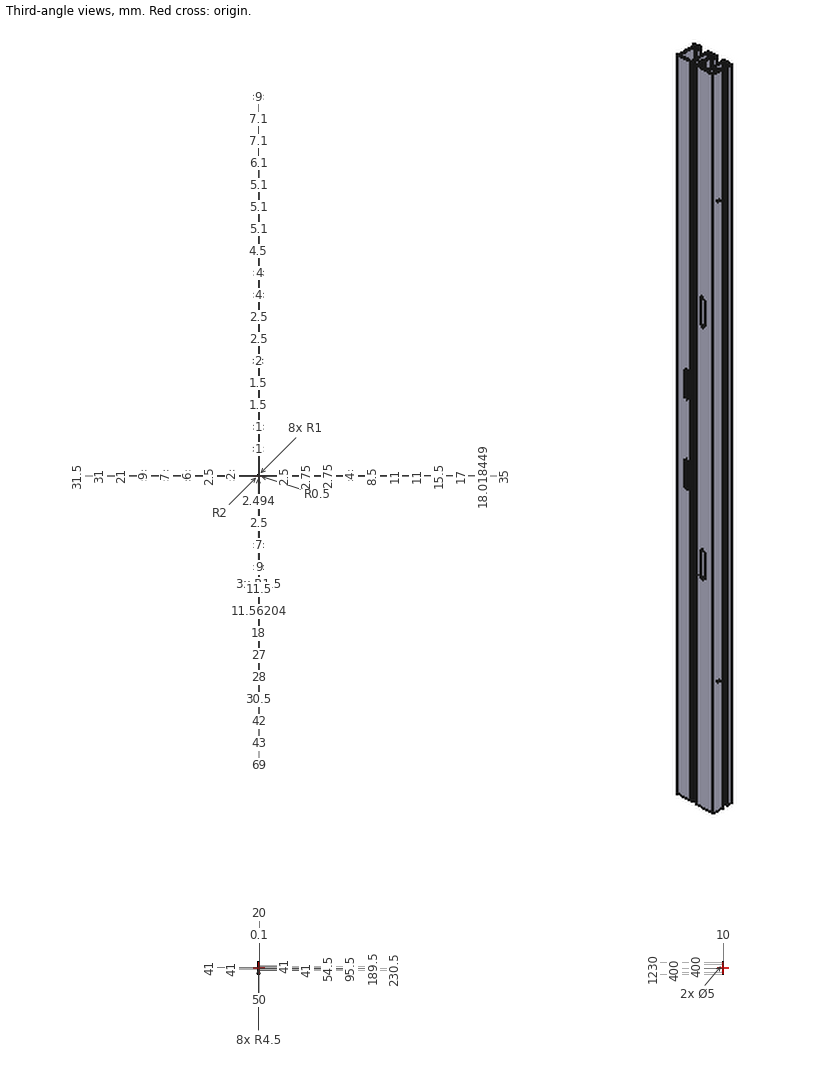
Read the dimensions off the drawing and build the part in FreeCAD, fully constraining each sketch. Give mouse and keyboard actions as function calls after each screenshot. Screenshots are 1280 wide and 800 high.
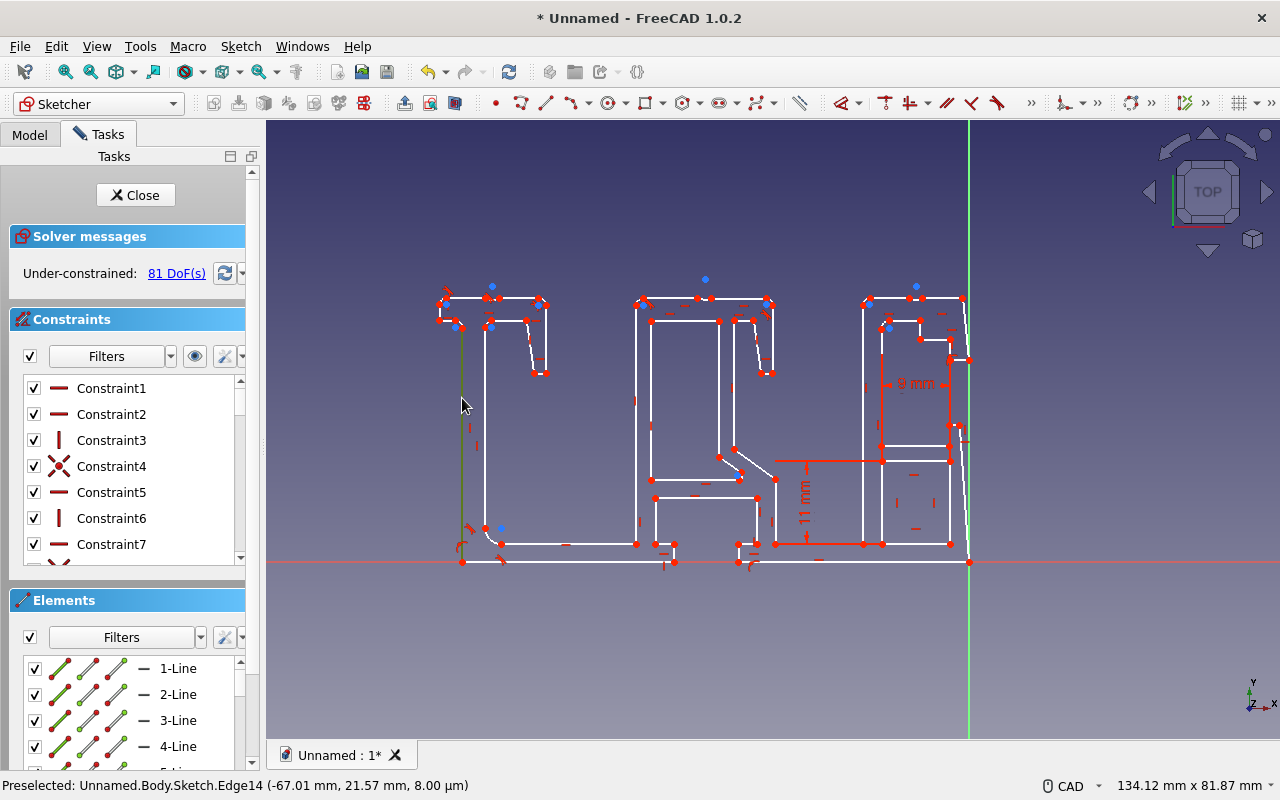
scroll(461, 323, up, 5)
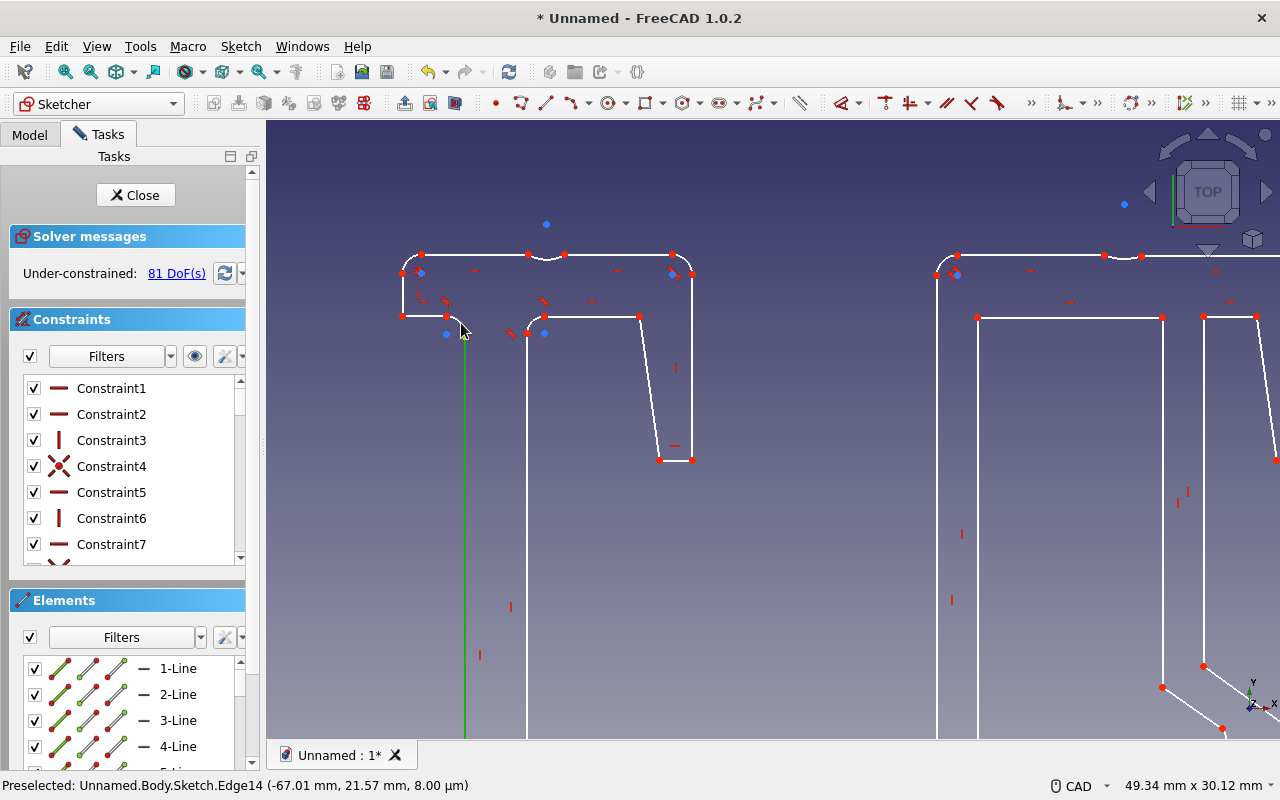
click(460, 323)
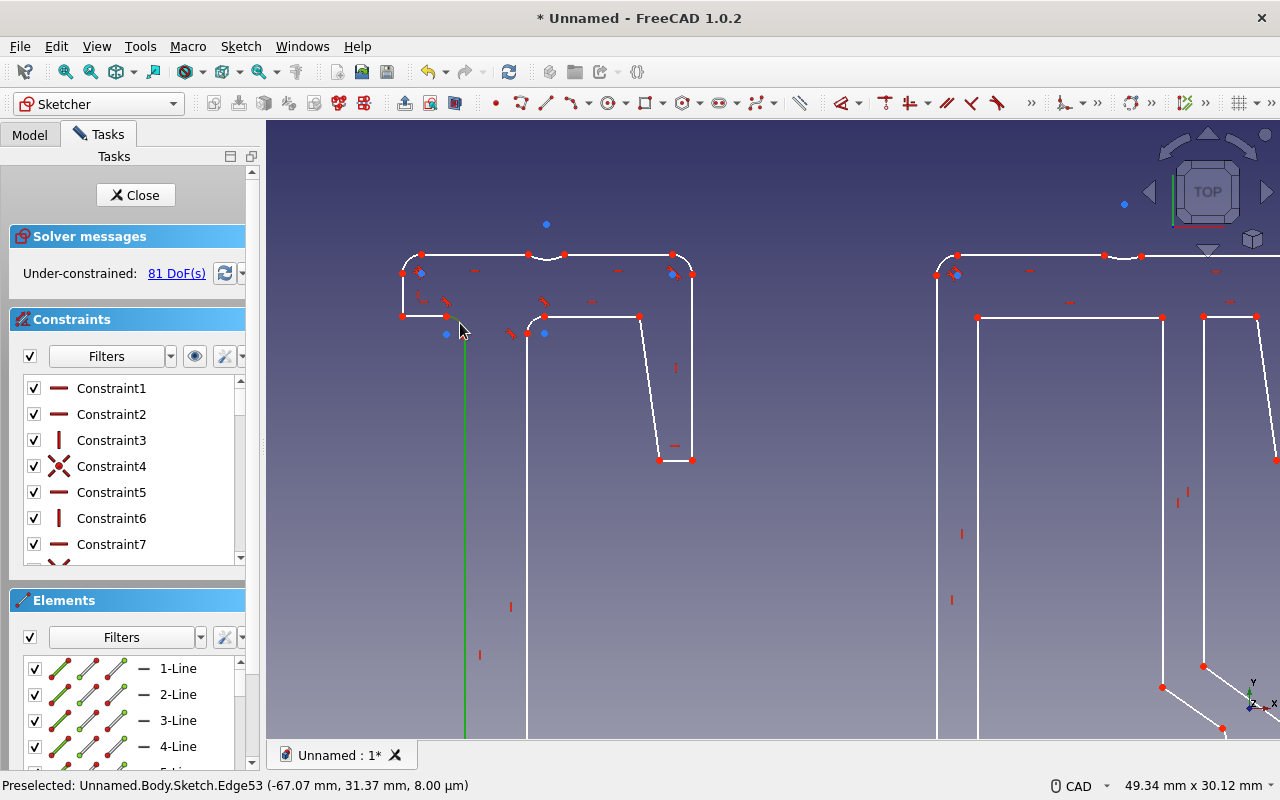
click(997, 104)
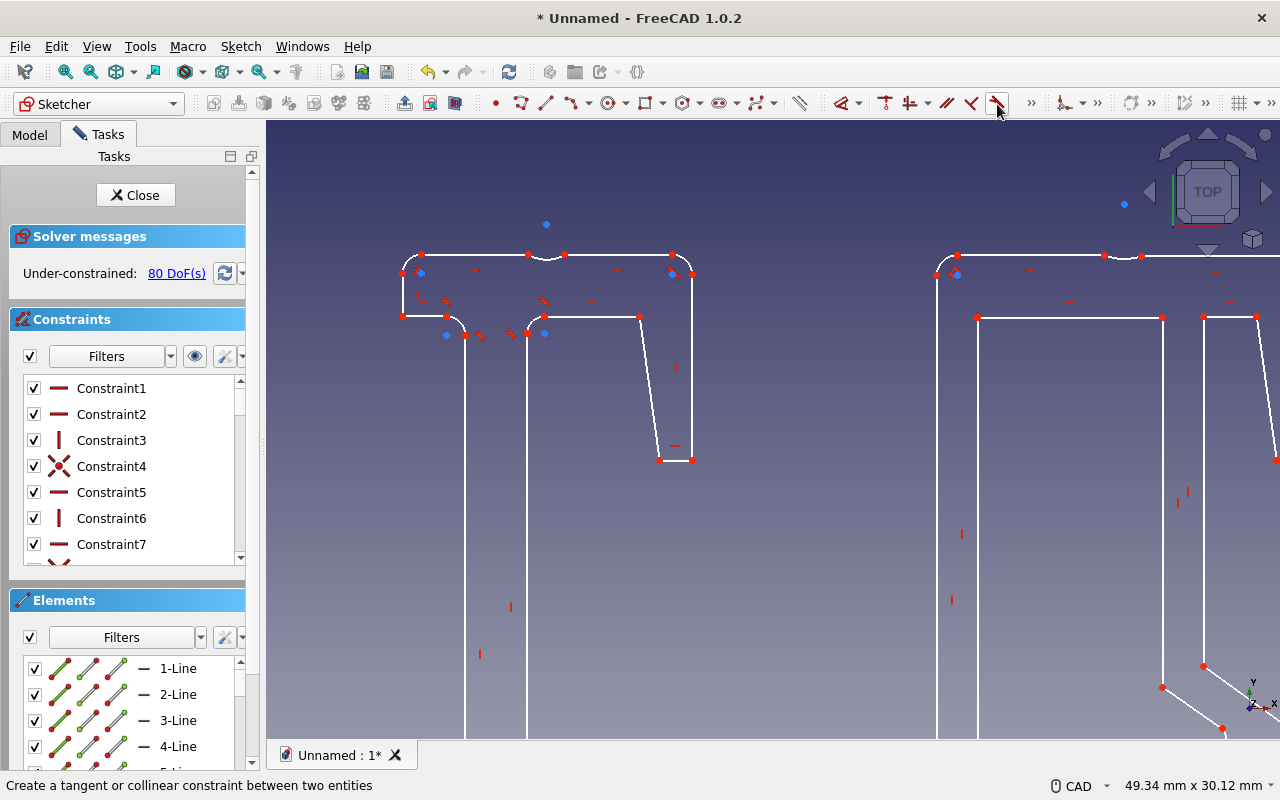
scroll(461, 323, down, 5)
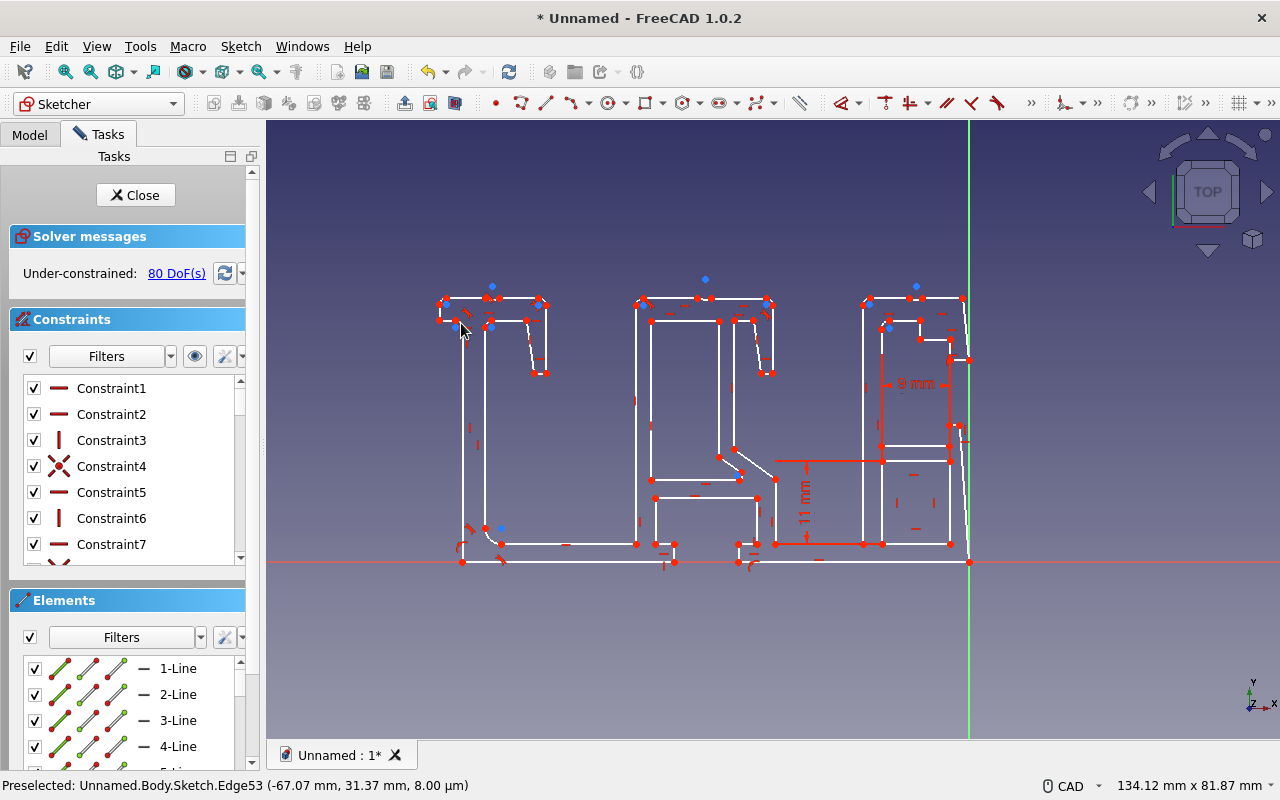
click(882, 411)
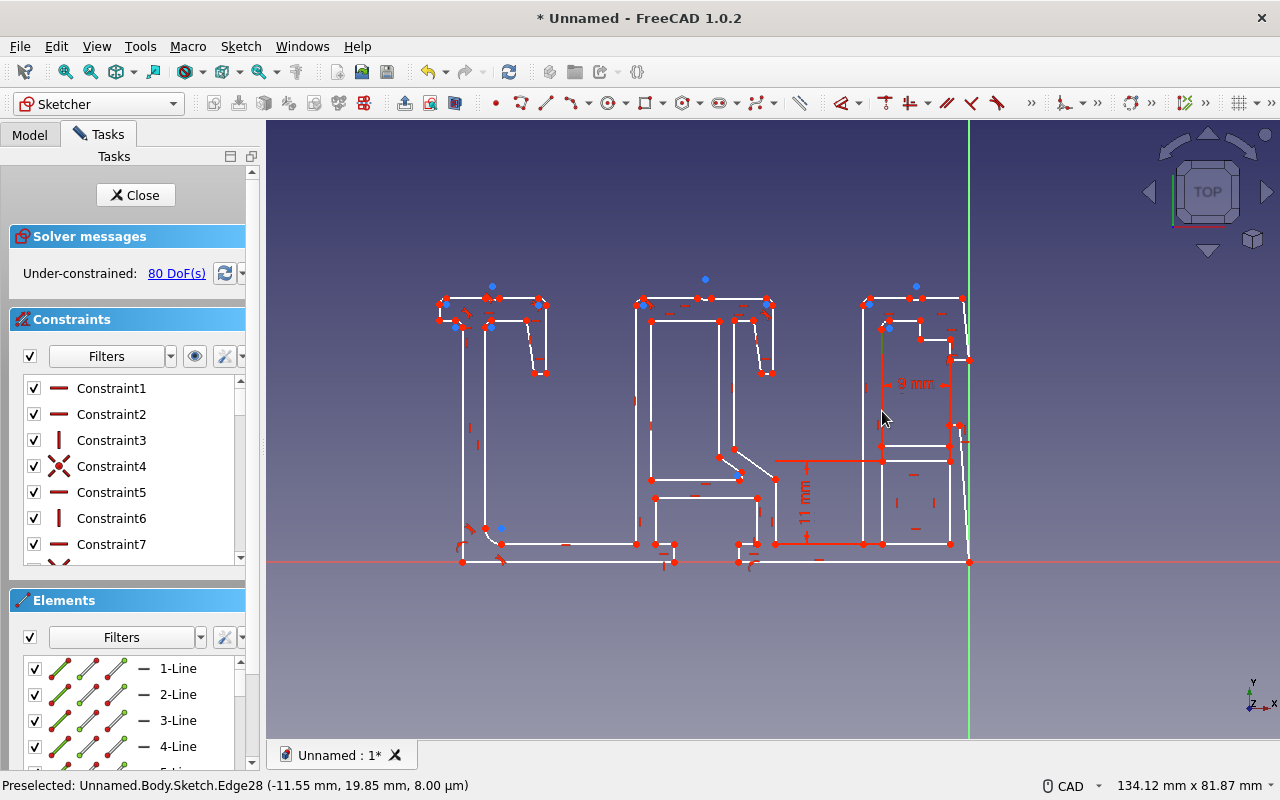
scroll(884, 323, up, 4)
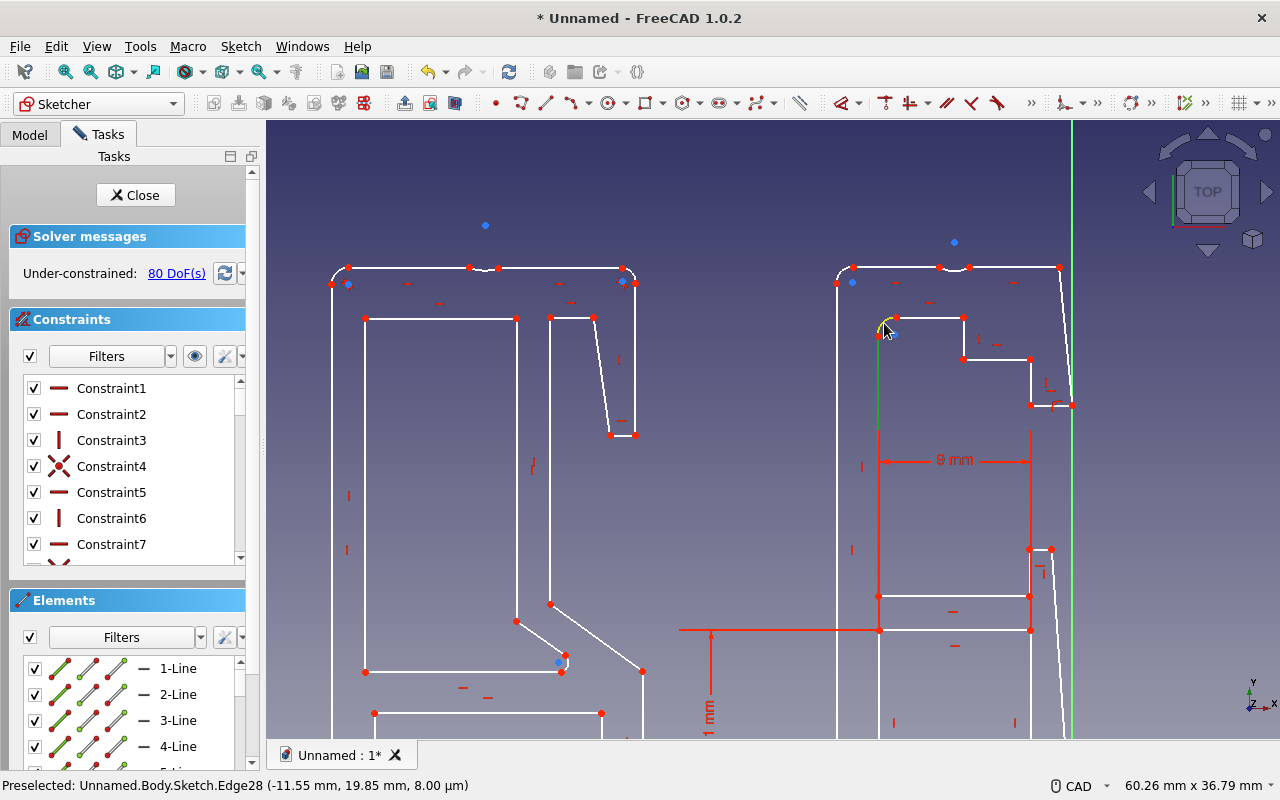
click(883, 323)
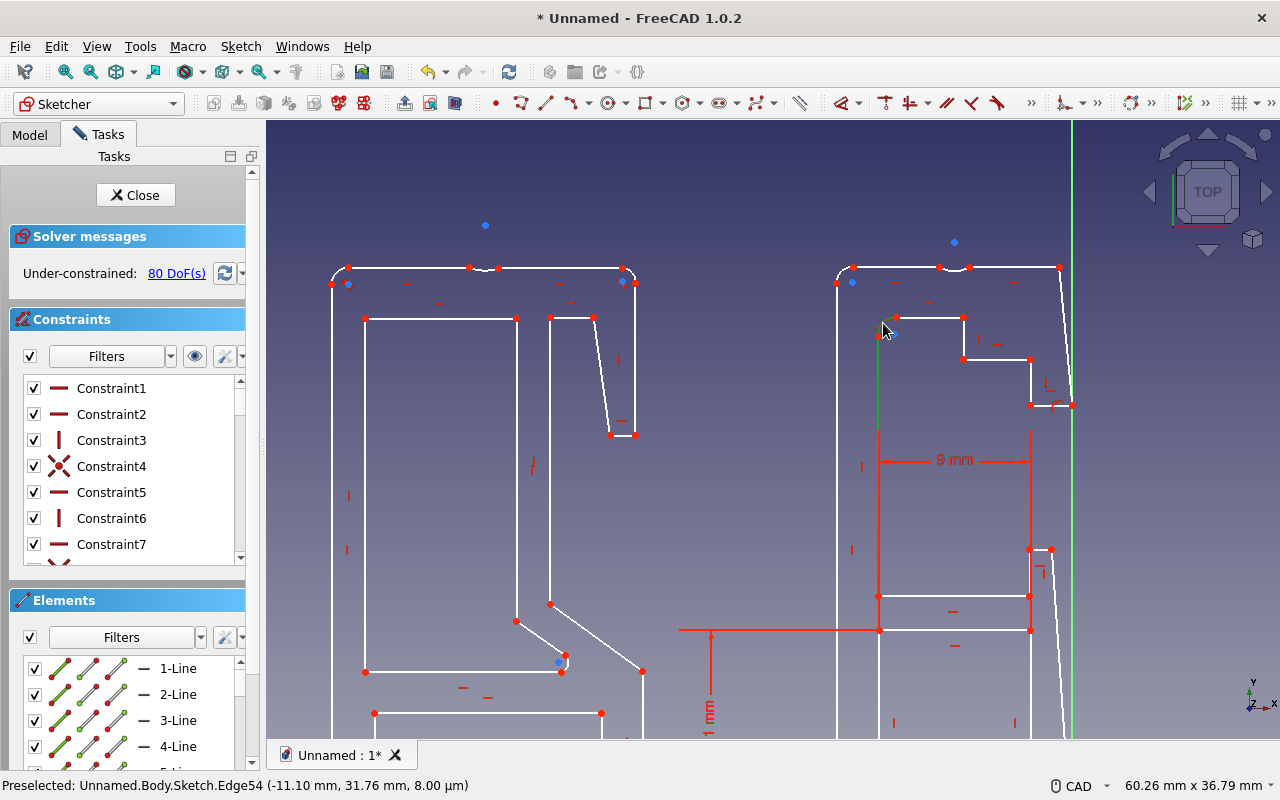
click(997, 104)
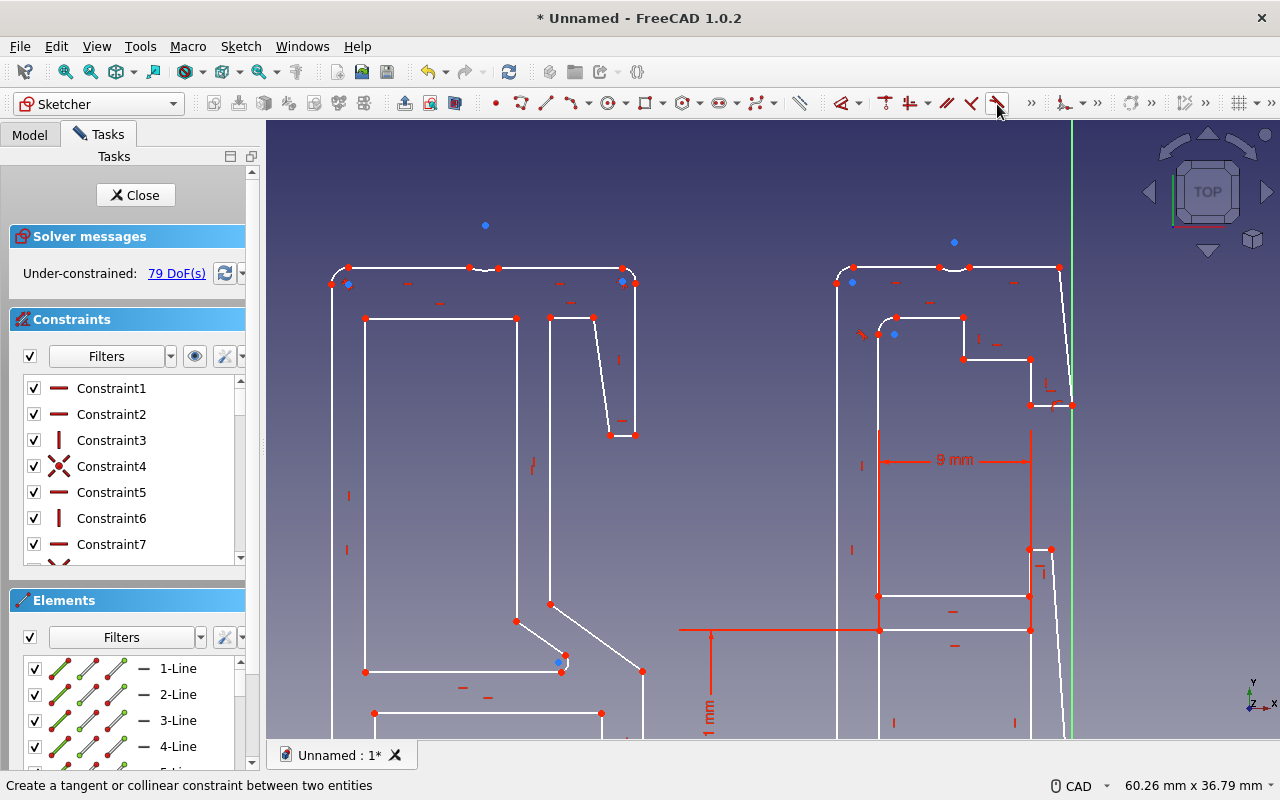
click(917, 318)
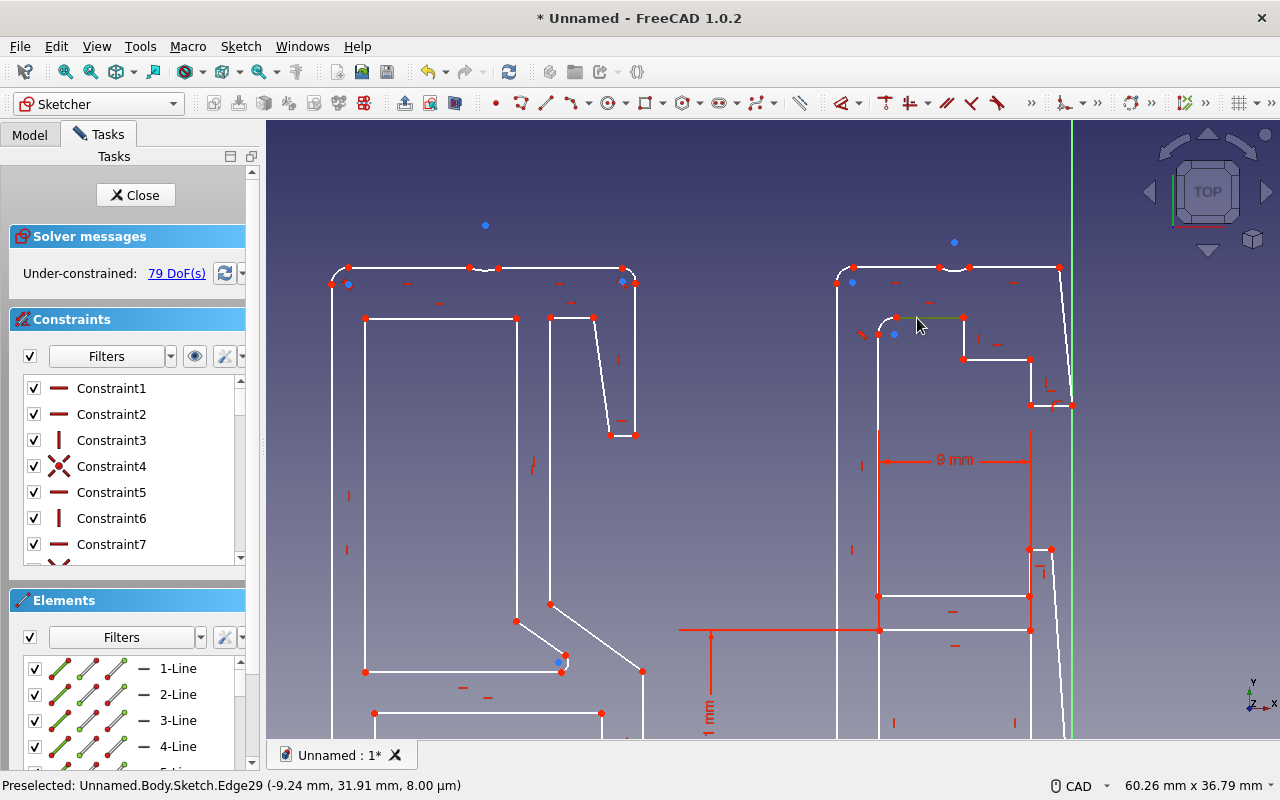
click(884, 322)